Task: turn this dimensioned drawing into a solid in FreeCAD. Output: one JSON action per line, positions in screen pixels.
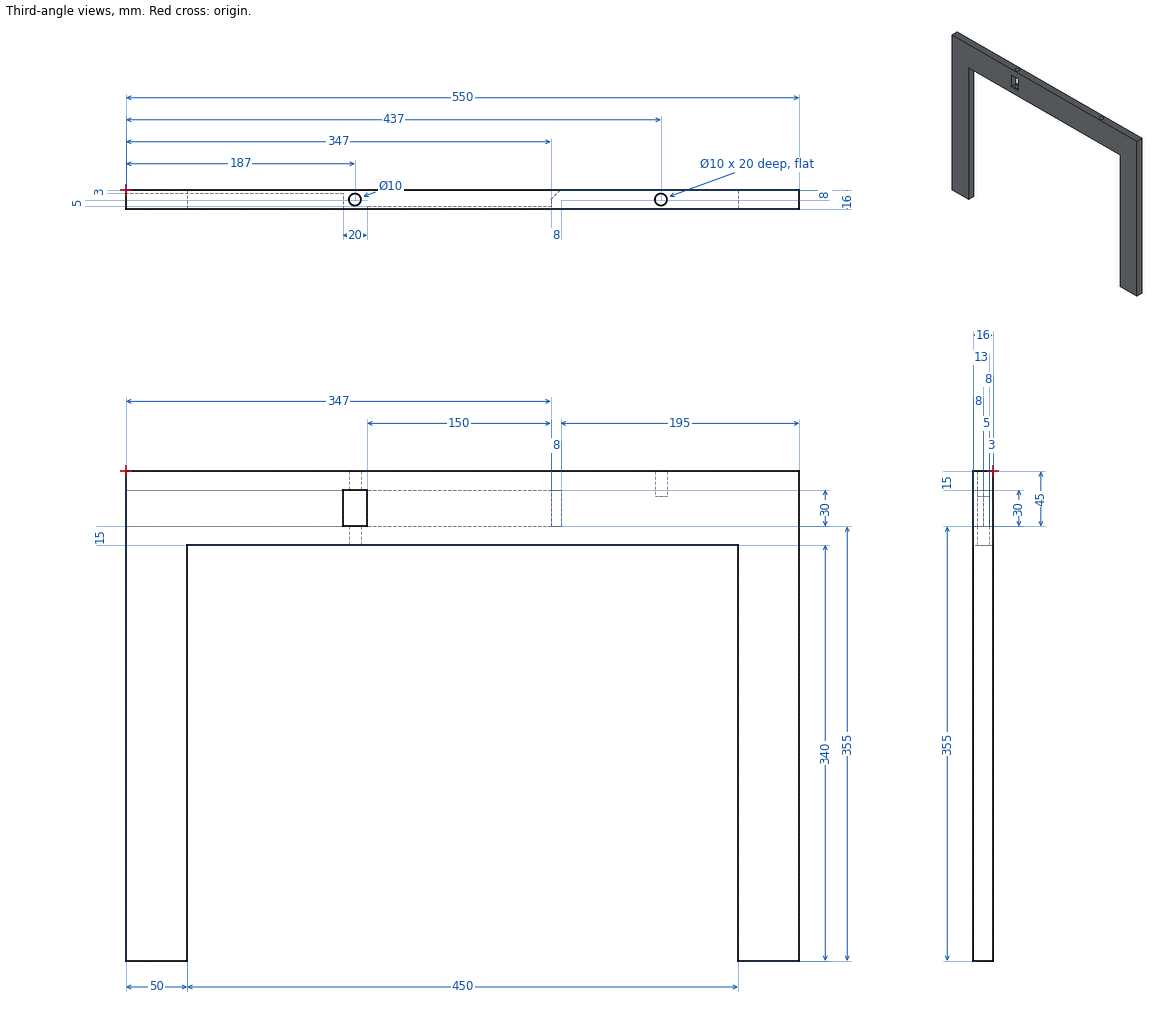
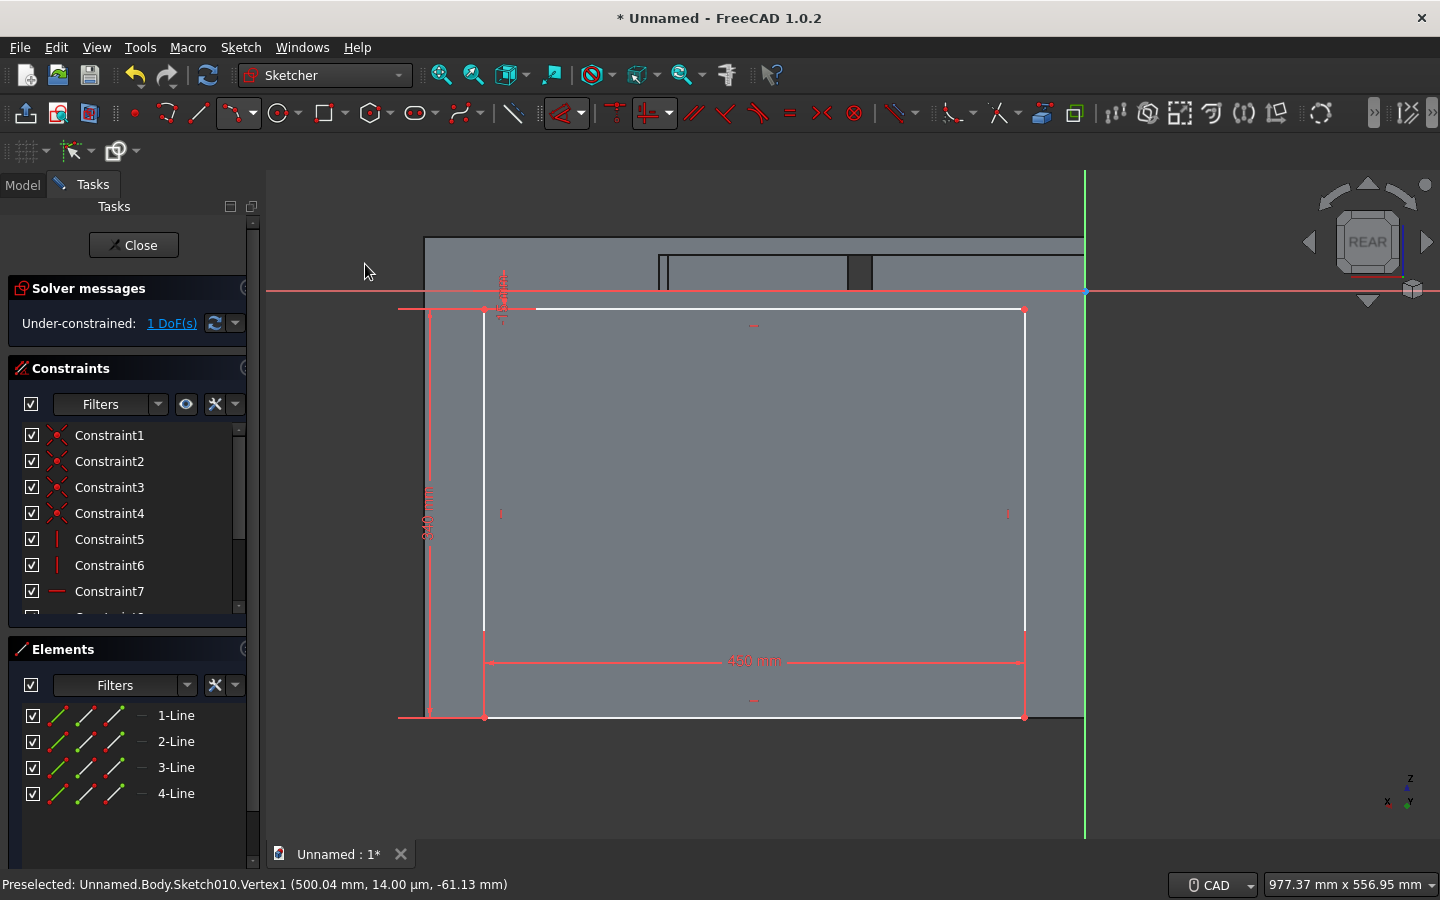
{"action": "left_click", "coordinate": [1025, 718]}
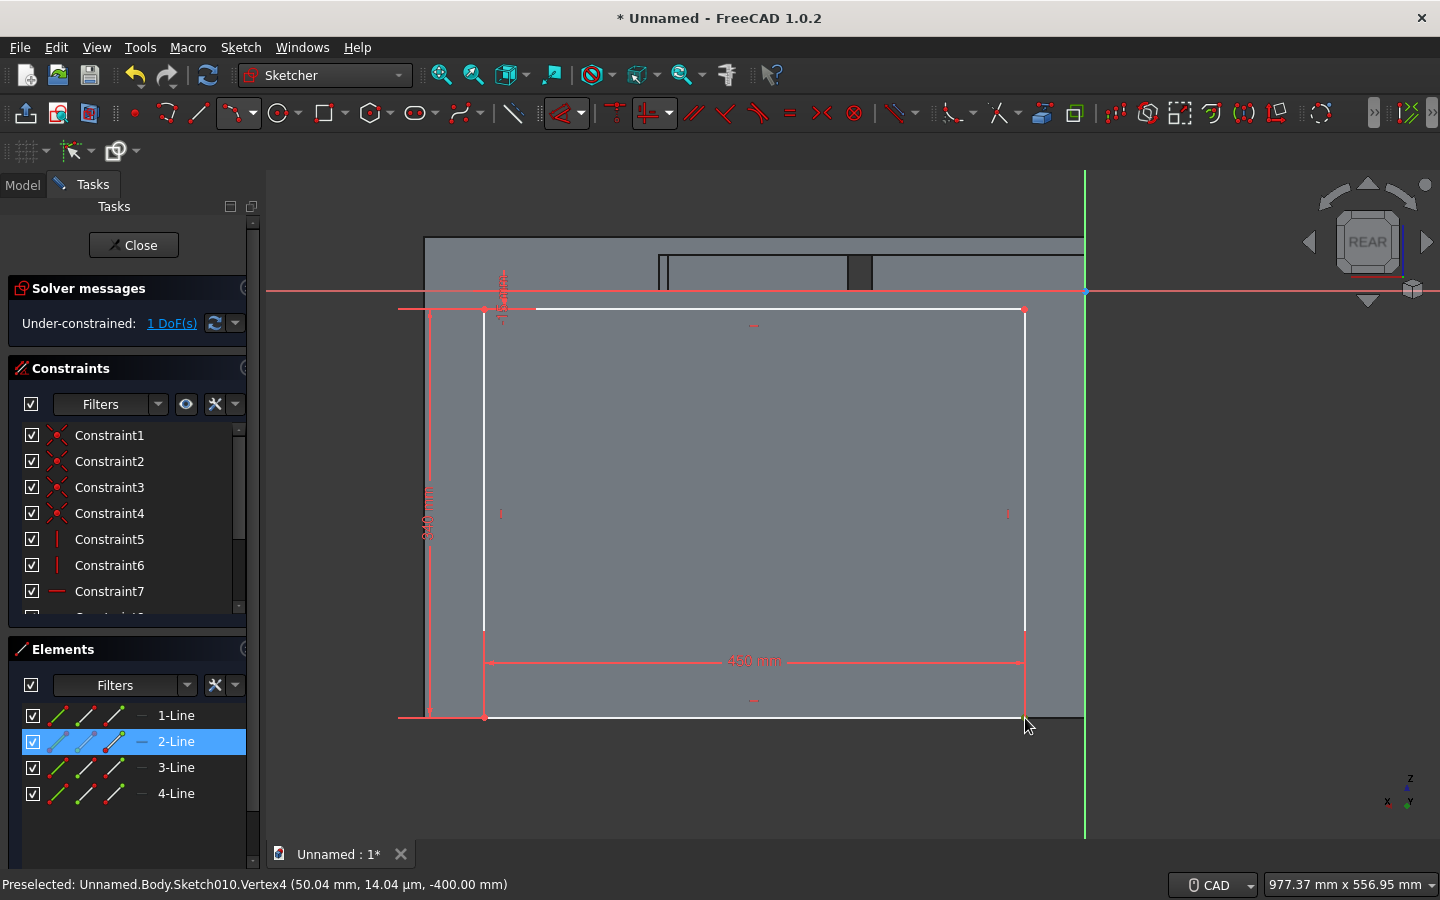
{"action": "left_click", "coordinate": [584, 114]}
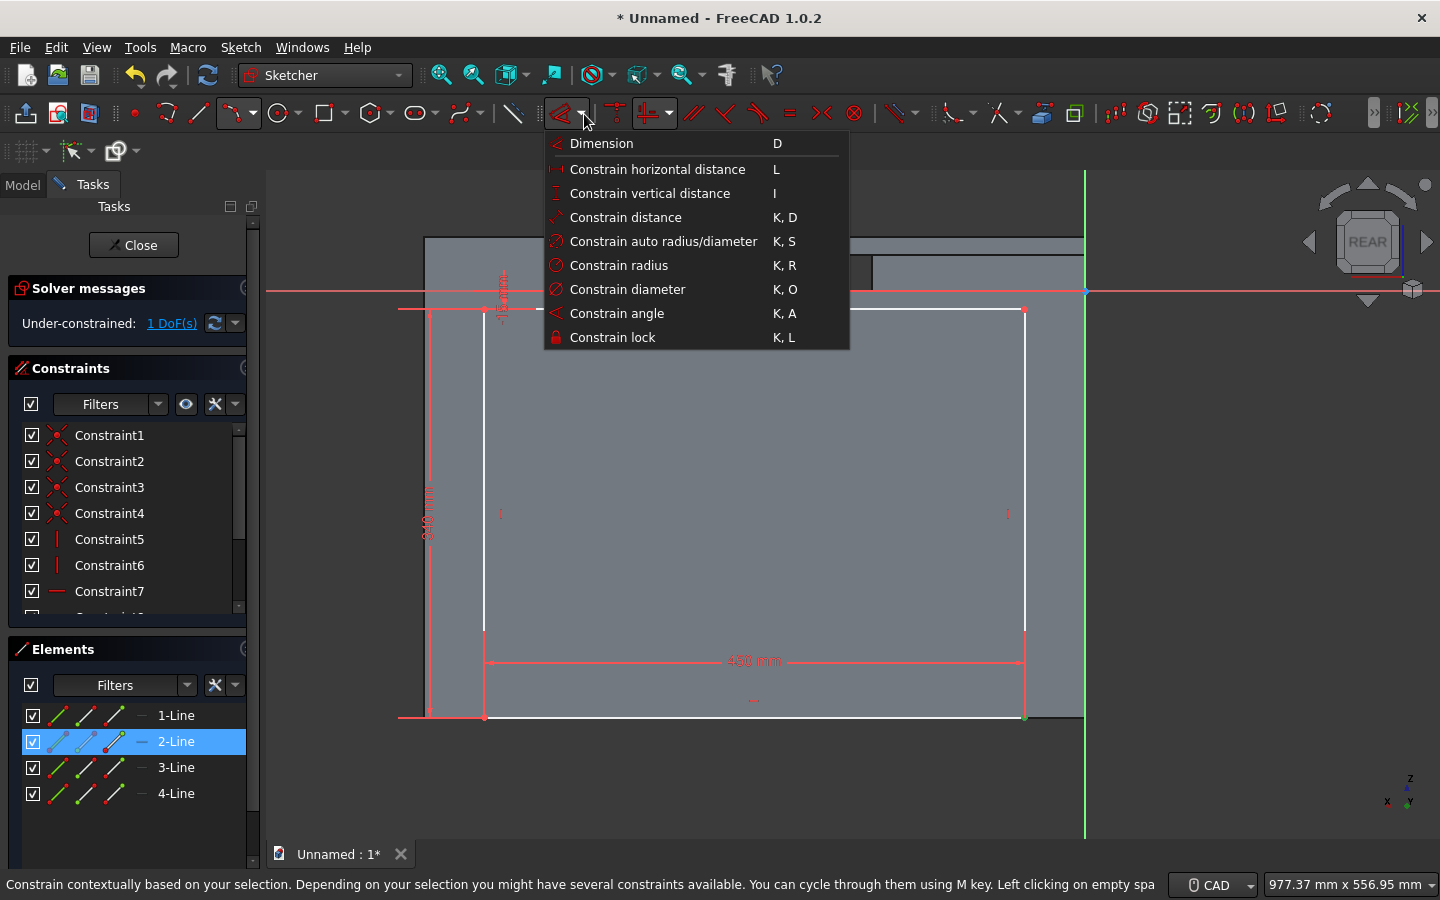
{"action": "left_click", "coordinate": [697, 169]}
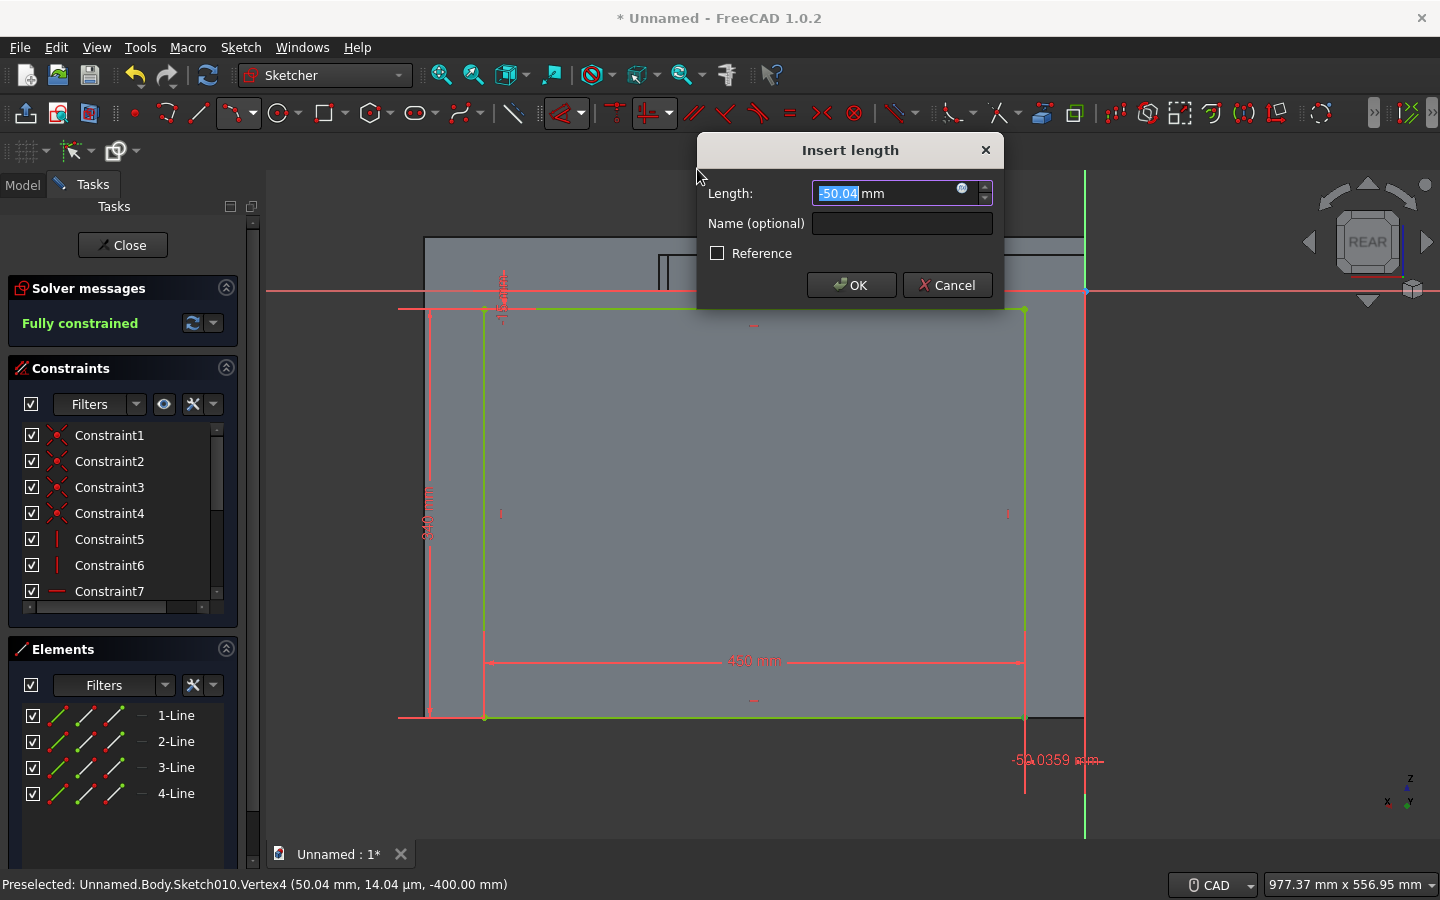
{"action": "type", "text": "-50"}
{"action": "key", "text": "Return"}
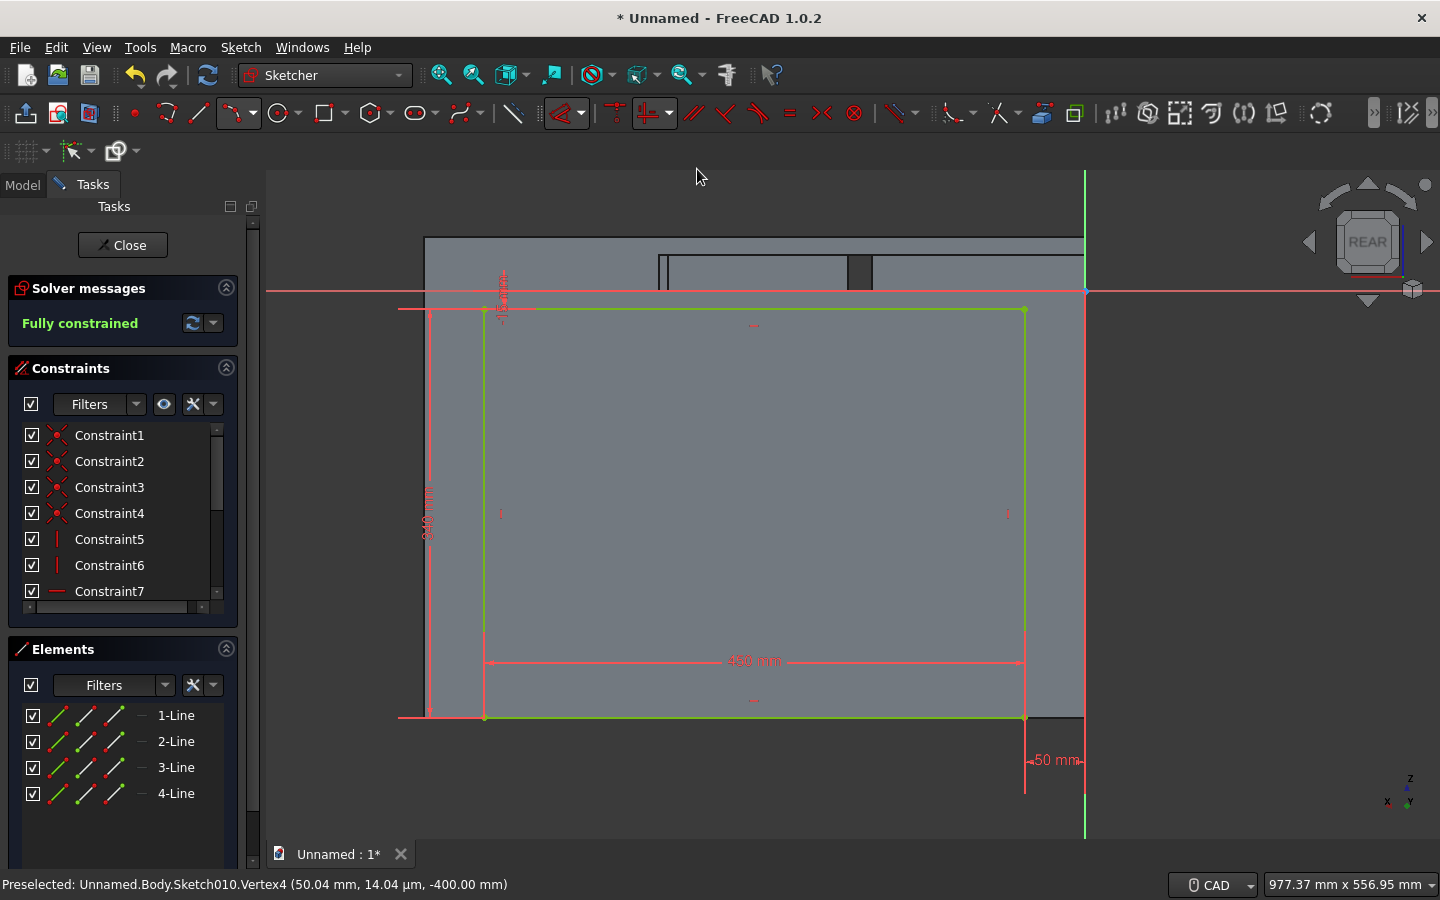
{"action": "left_click", "coordinate": [123, 245]}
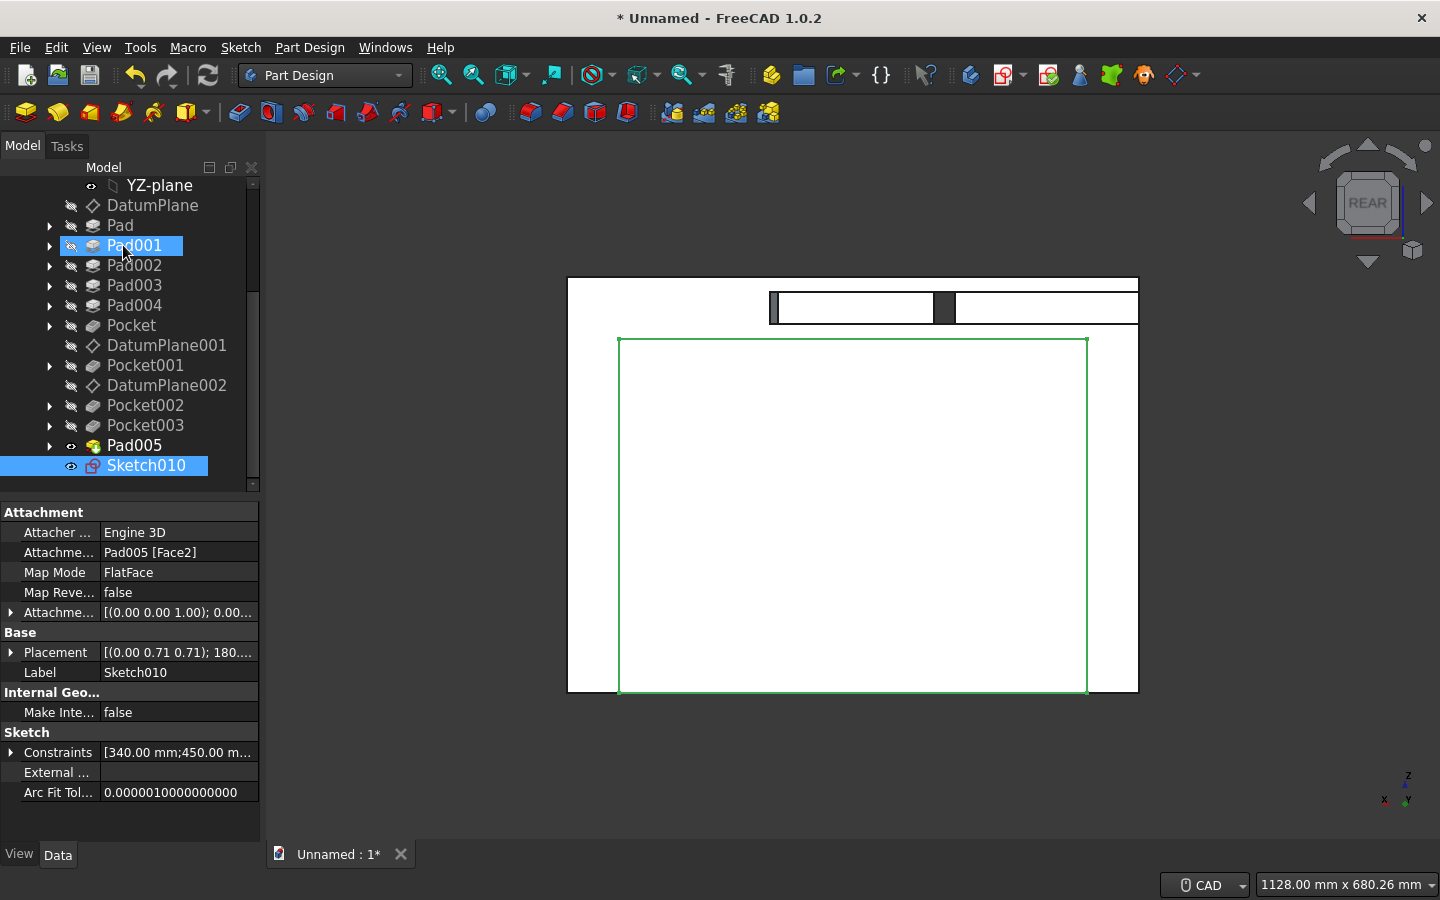
{"action": "left_click", "coordinate": [240, 112]}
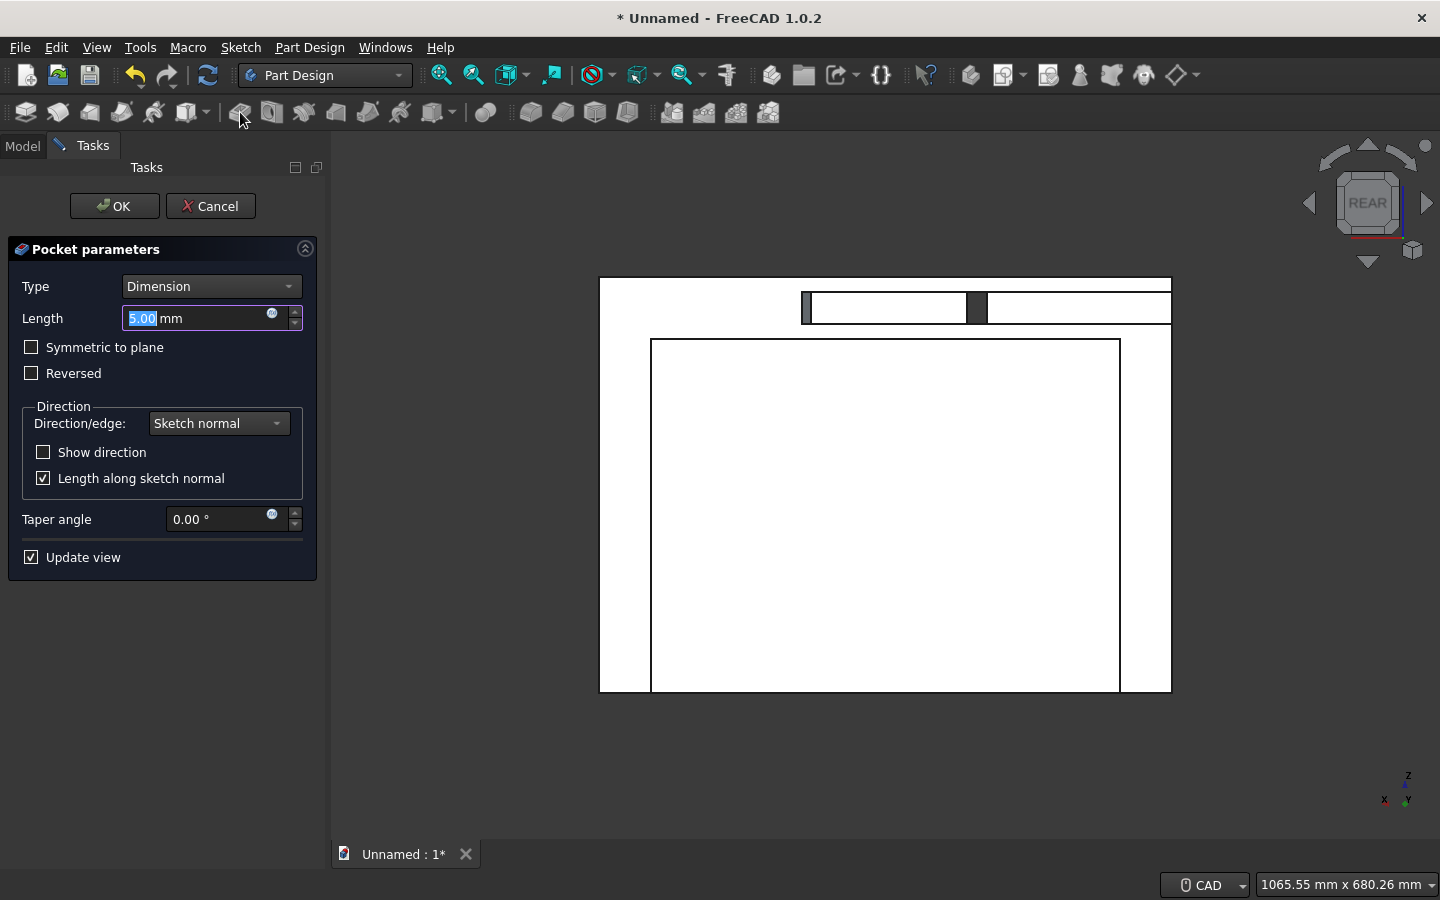
{"action": "left_click", "coordinate": [212, 286]}